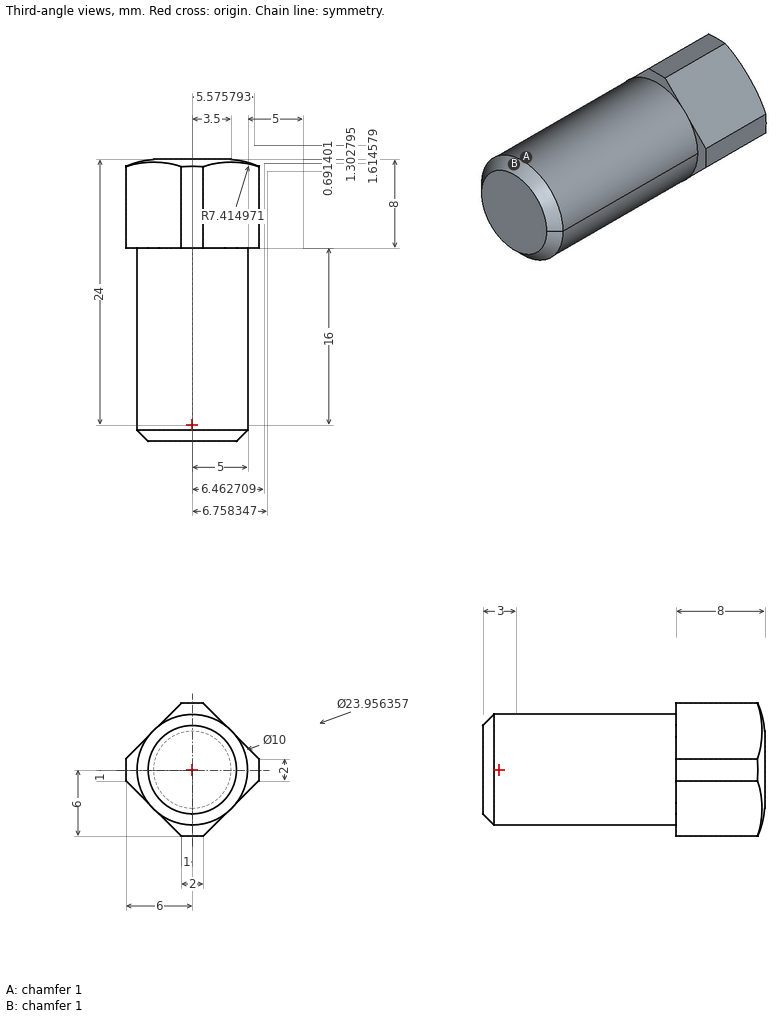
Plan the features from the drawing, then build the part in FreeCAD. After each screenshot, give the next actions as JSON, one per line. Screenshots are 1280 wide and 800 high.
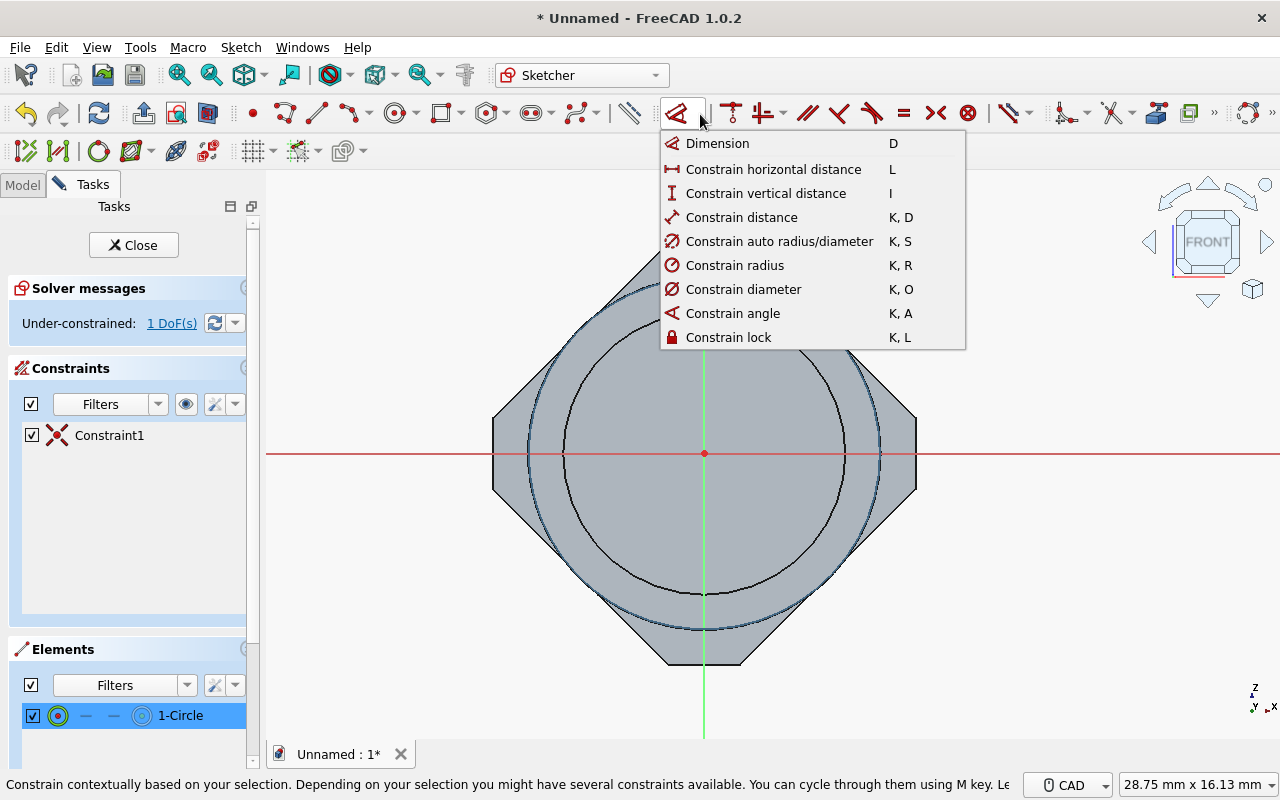
{"action": "left_click", "coordinate": [813, 289]}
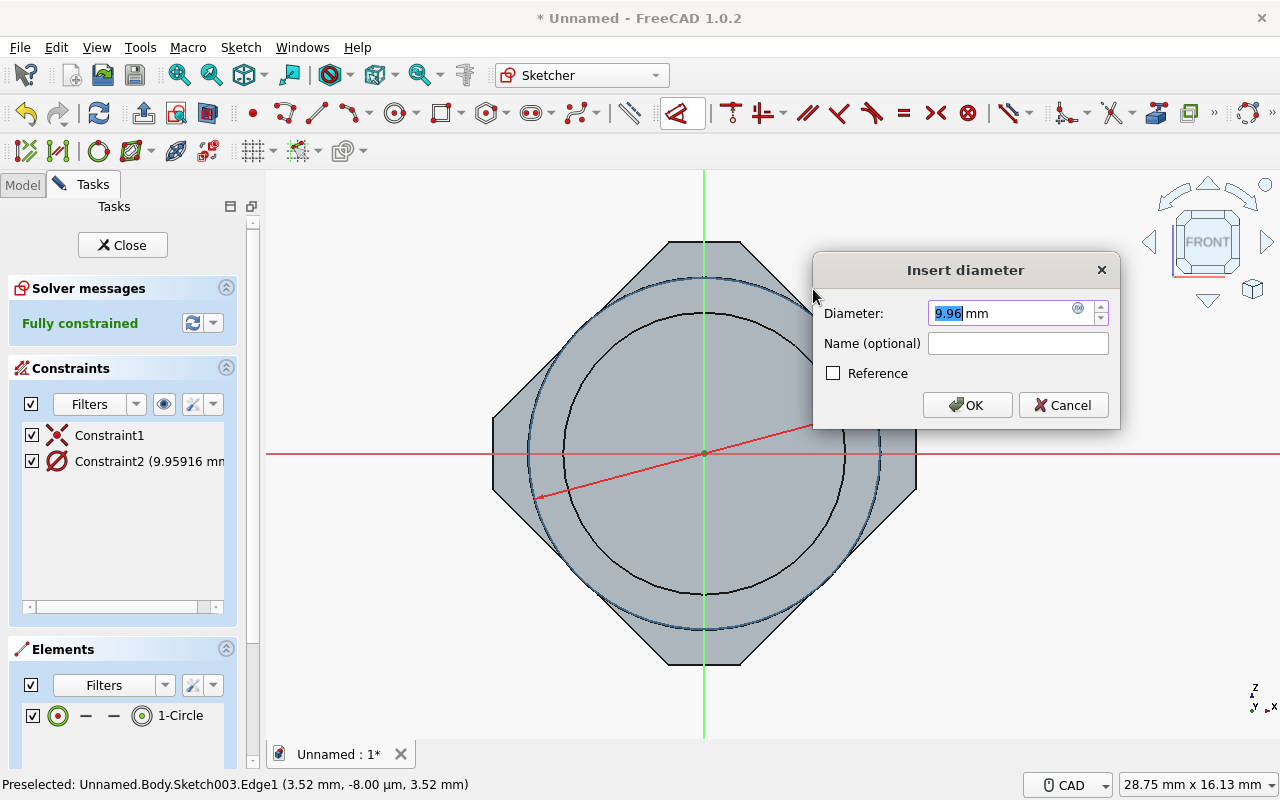
{"action": "type", "text": "10"}
{"action": "key", "text": "Return"}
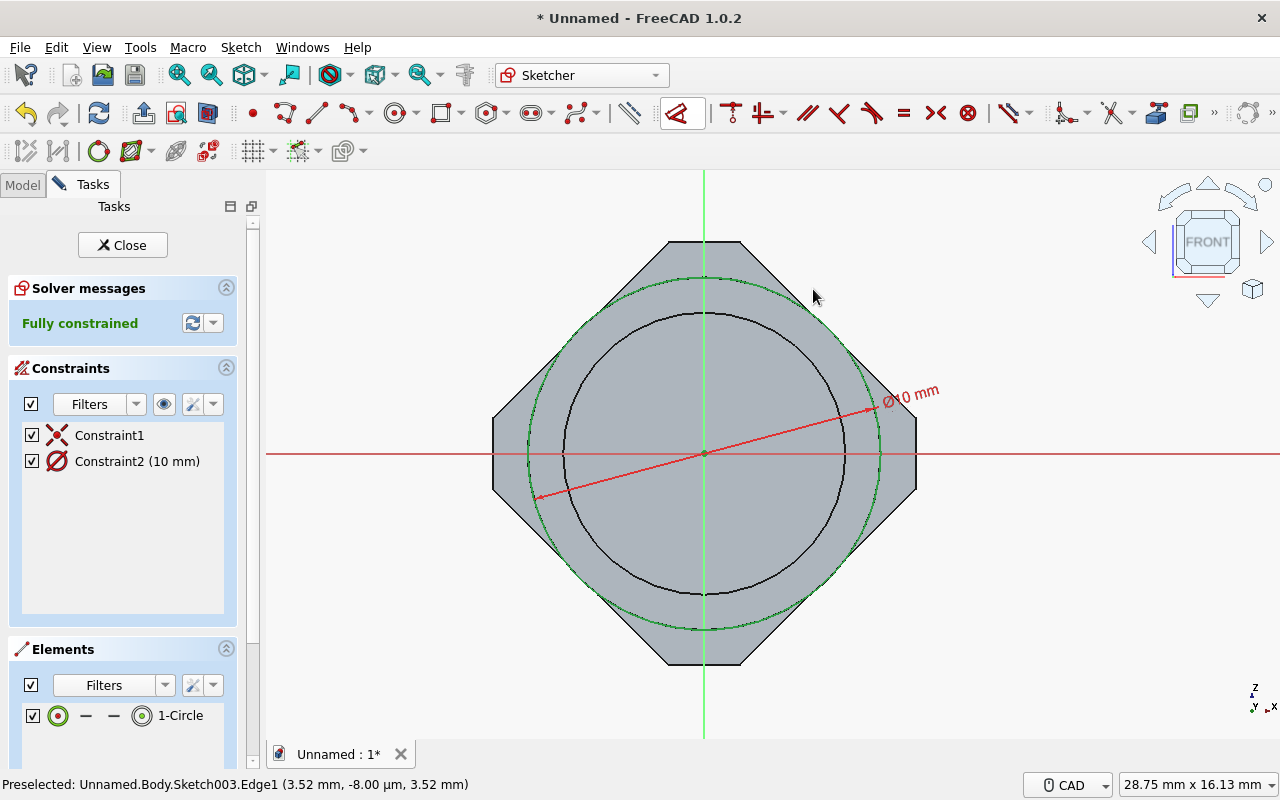
{"action": "left_click", "coordinate": [123, 245]}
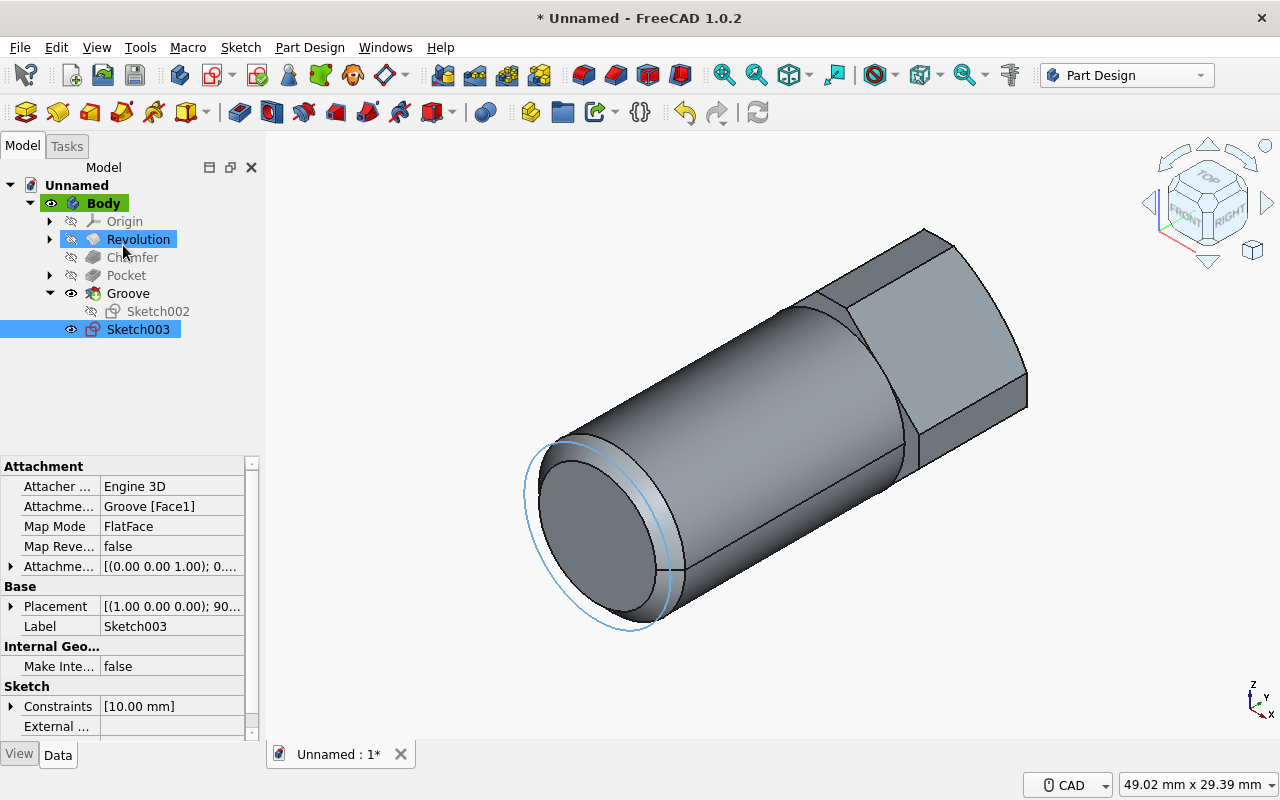
{"action": "left_click", "coordinate": [26, 112]}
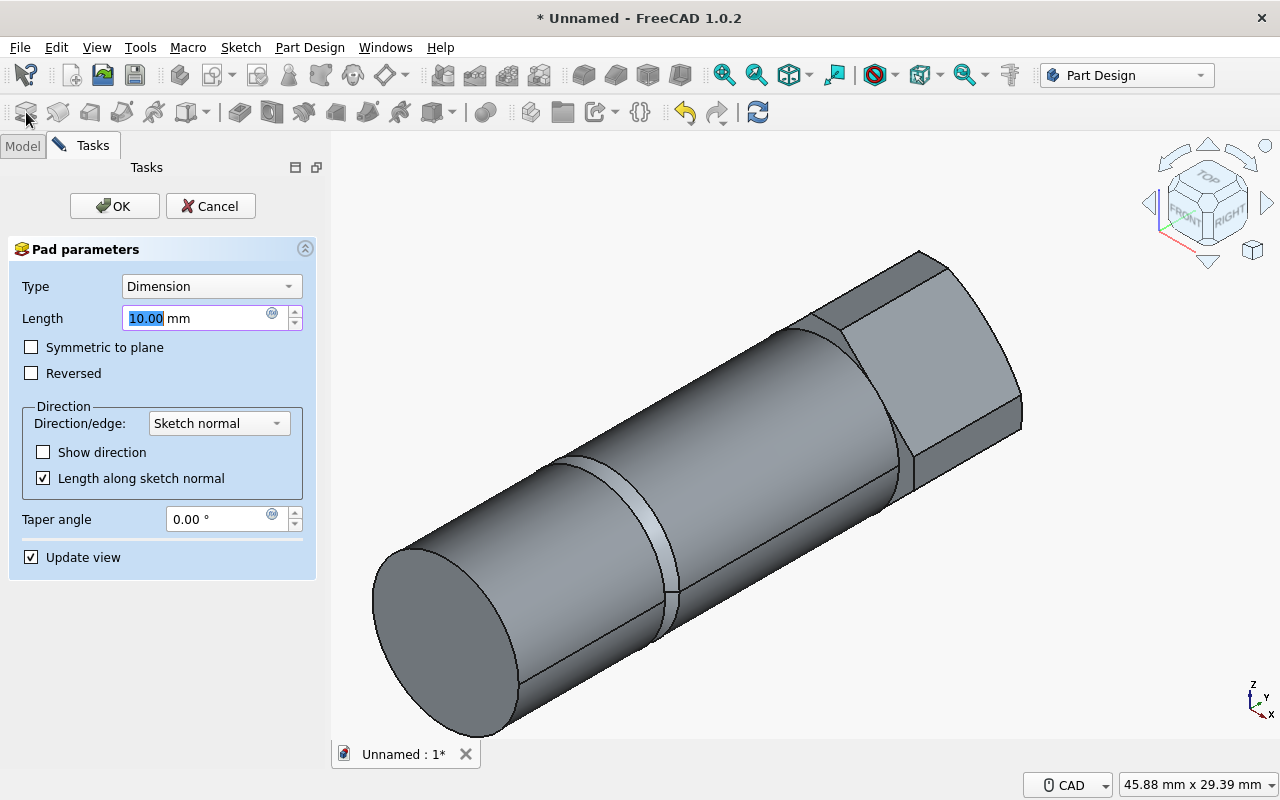
{"action": "type", "text": "3"}
{"action": "key", "text": "Tab"}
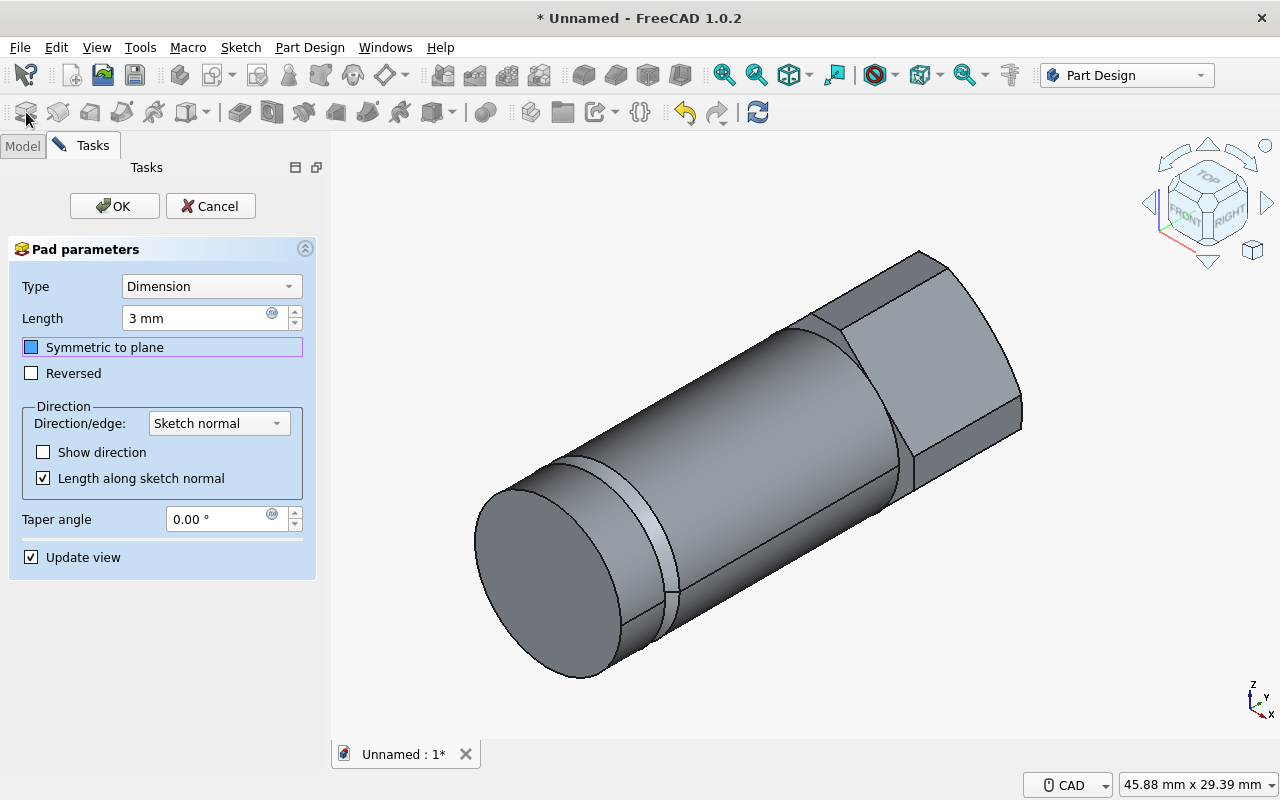
{"action": "left_click", "coordinate": [30, 347]}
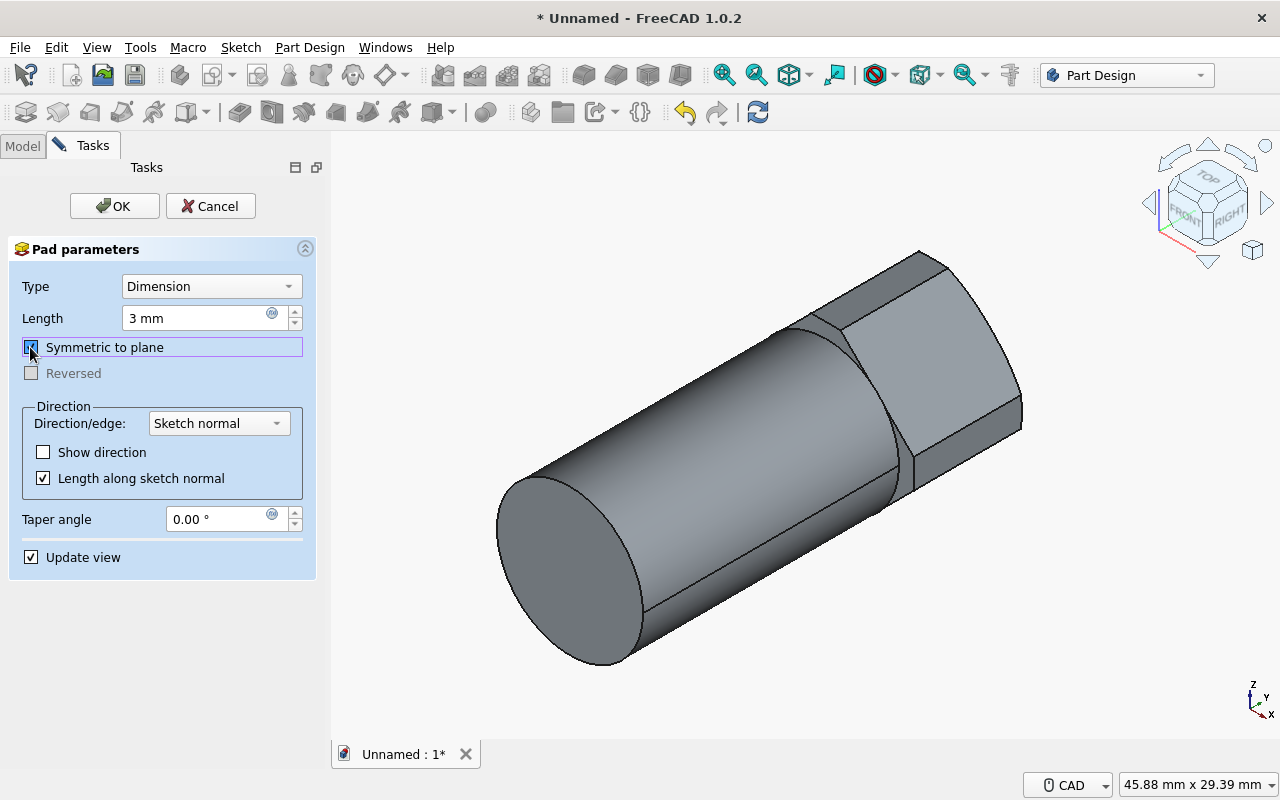
{"action": "left_click", "coordinate": [115, 206]}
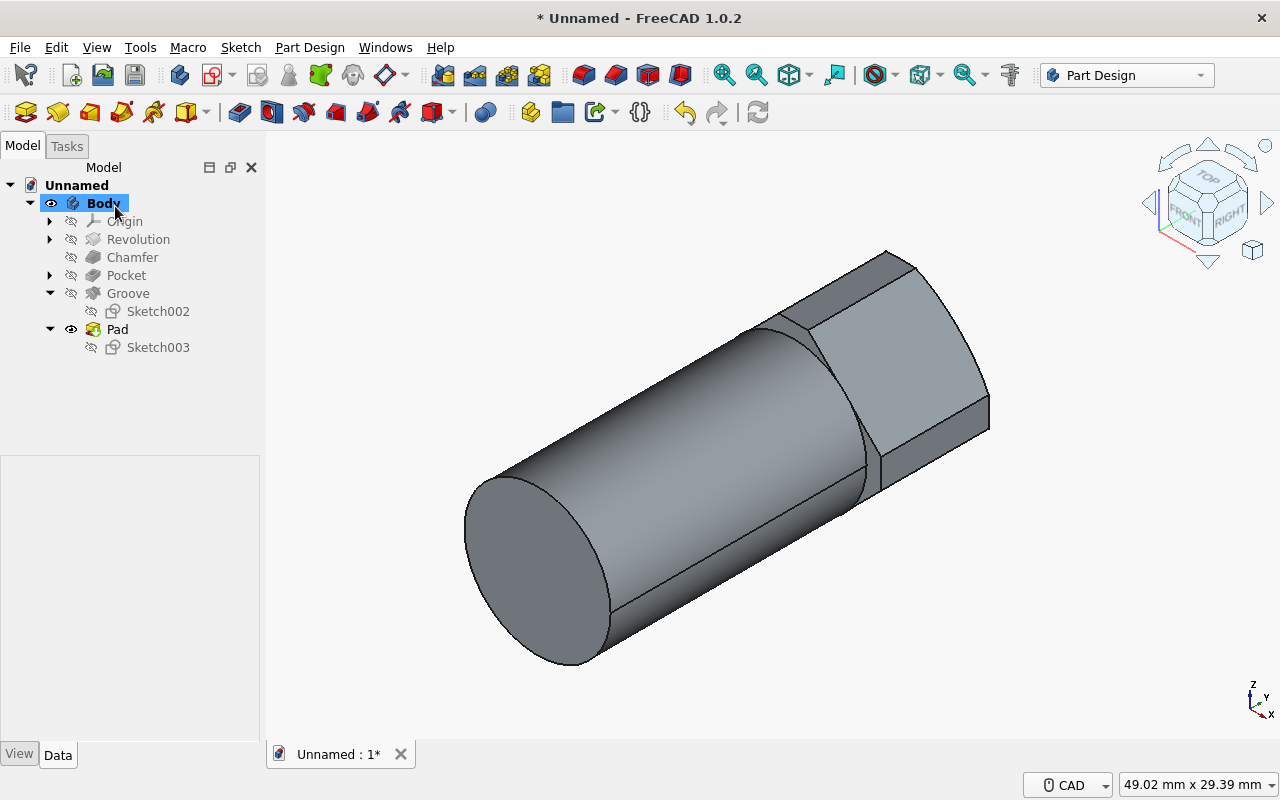
{"action": "left_click", "coordinate": [515, 477]}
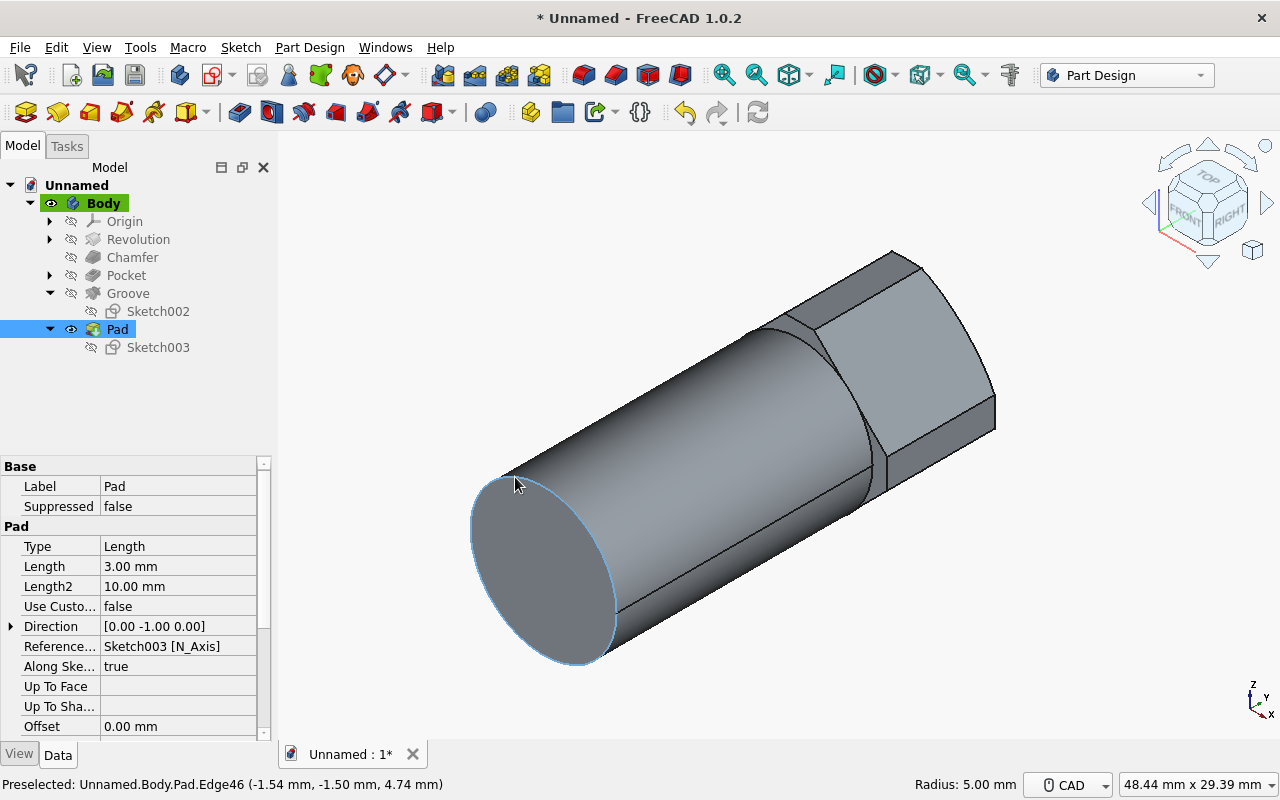
{"action": "left_click", "coordinate": [616, 76]}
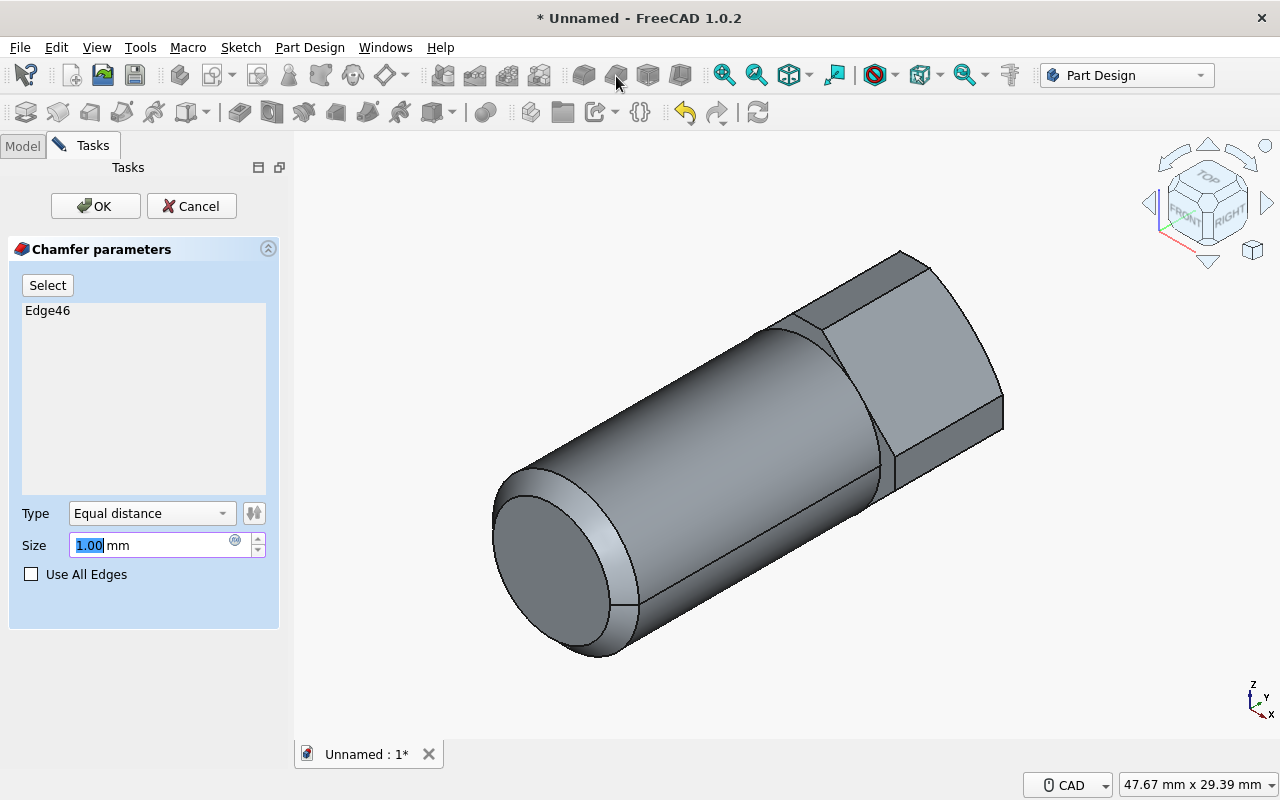
{"action": "type", "text": "1"}
{"action": "key", "text": "Tab"}